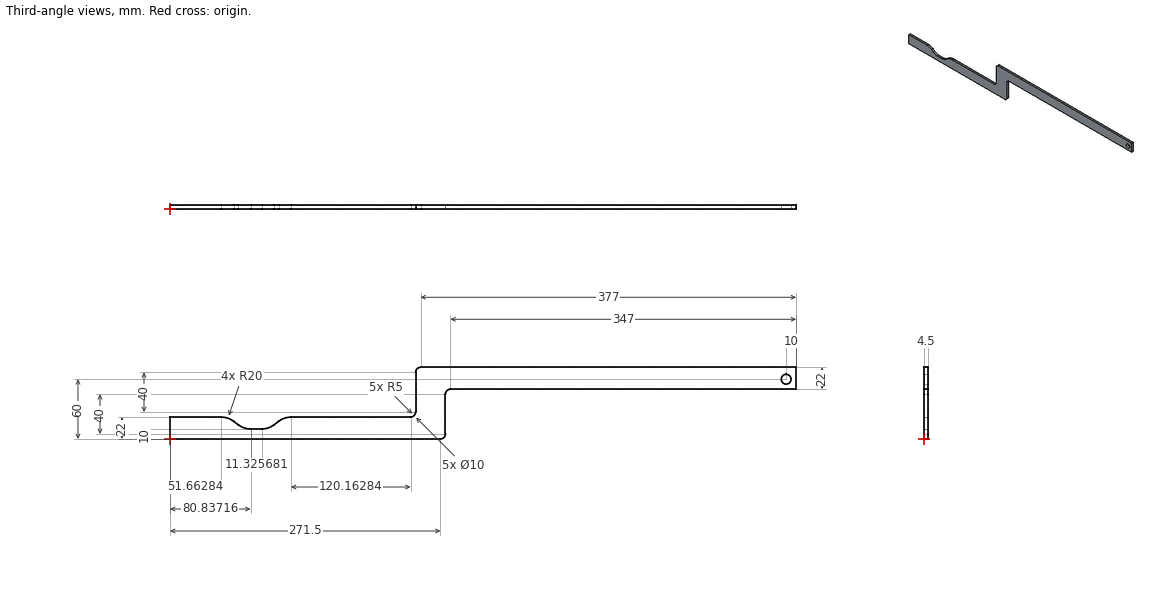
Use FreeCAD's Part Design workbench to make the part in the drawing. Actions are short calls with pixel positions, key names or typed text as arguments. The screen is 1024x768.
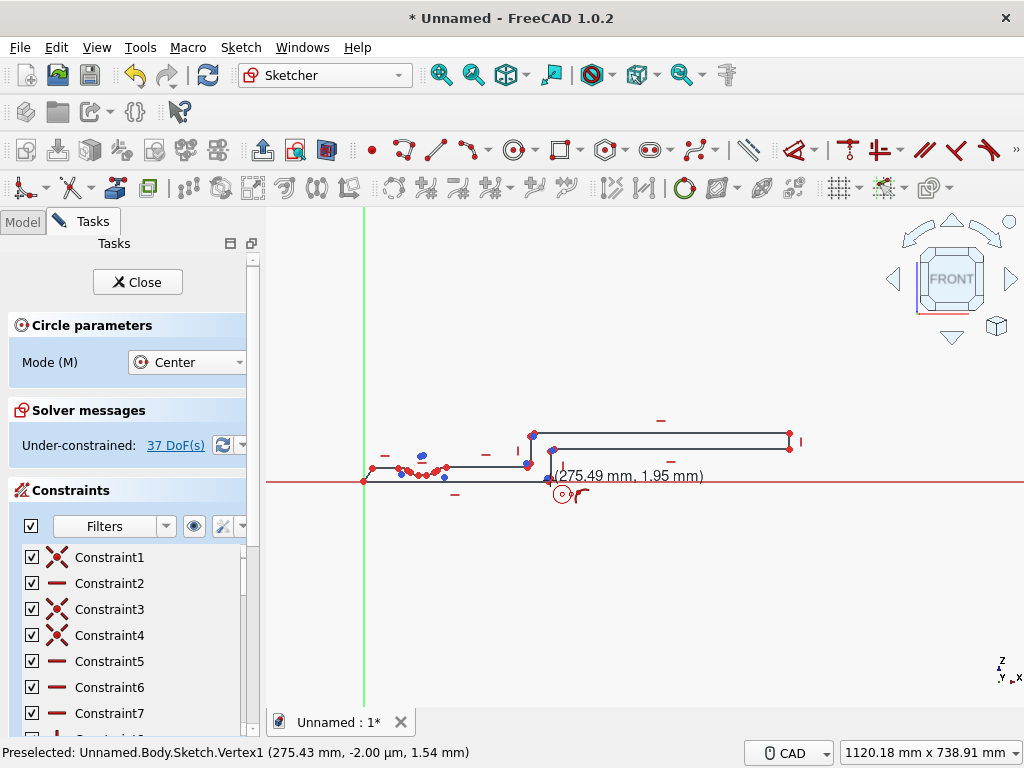
scroll(782, 441, up, 10)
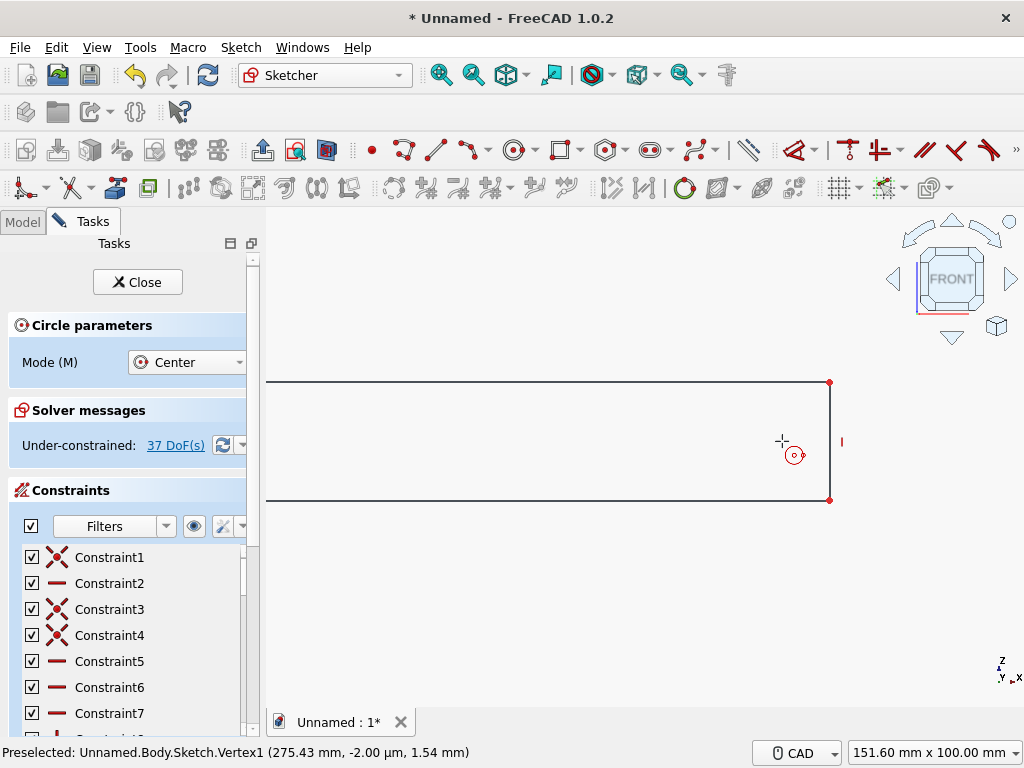
scroll(783, 441, down, 10)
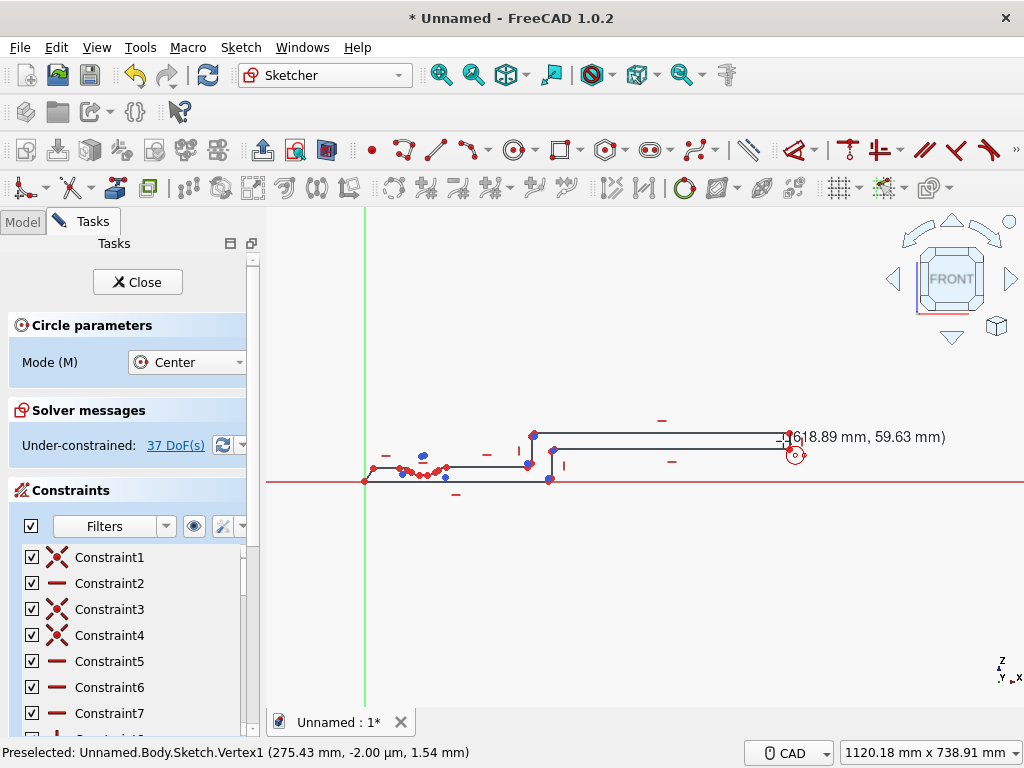
scroll(783, 441, up, 5)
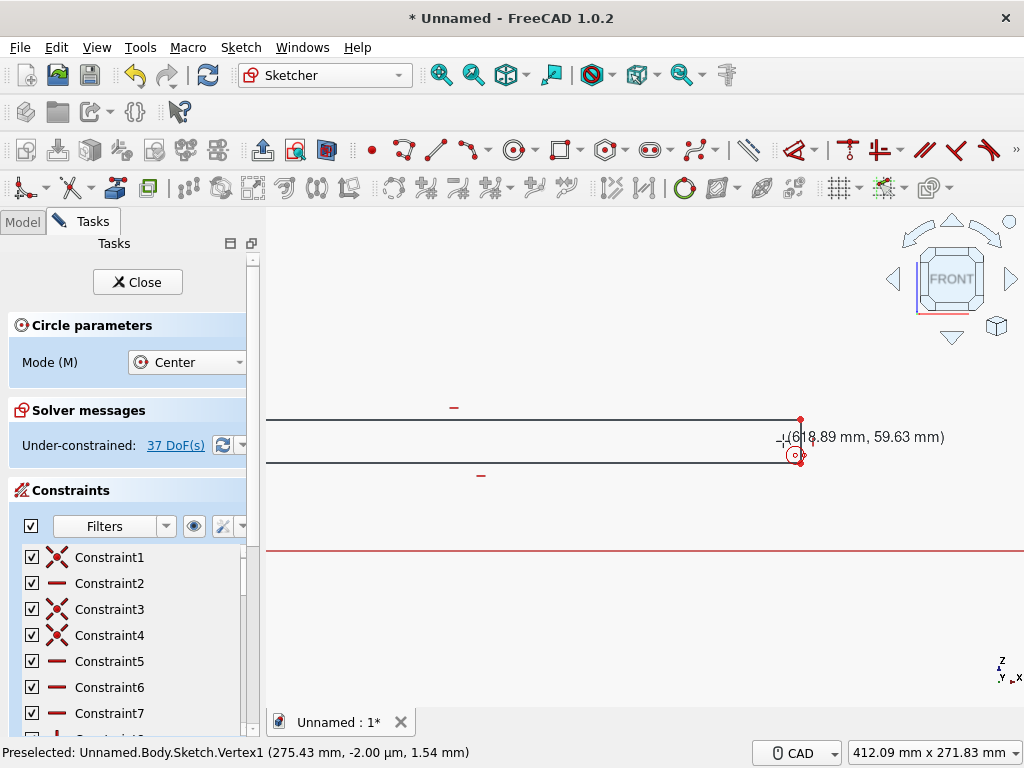
click(783, 441)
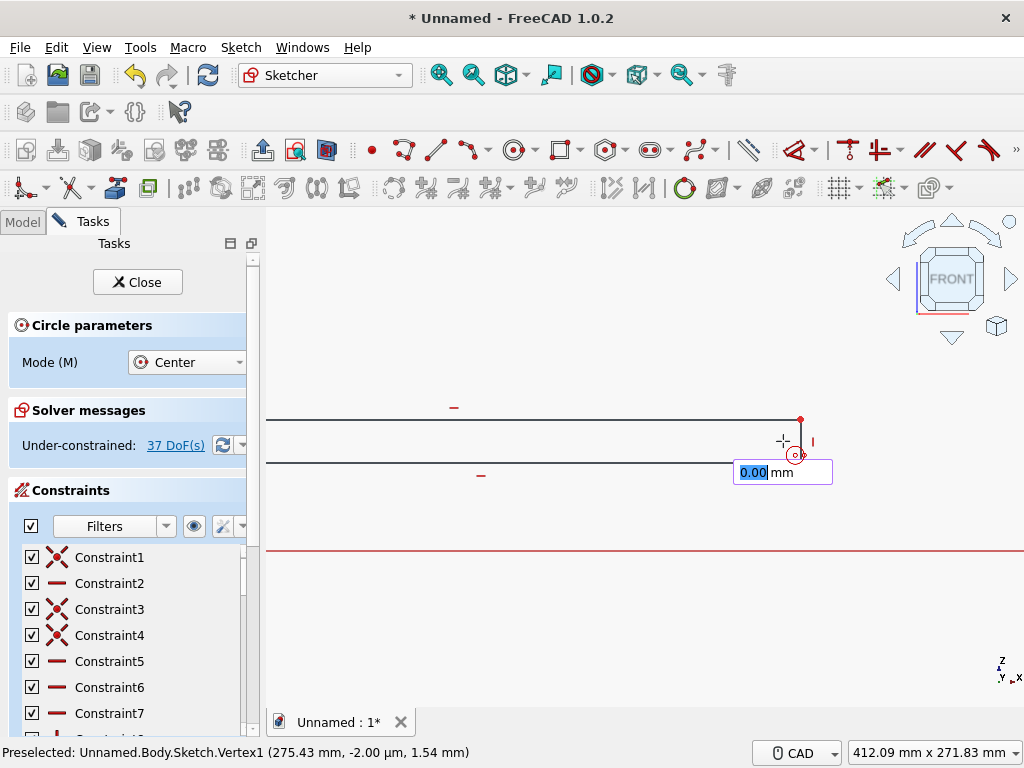
scroll(776, 434, up, 3)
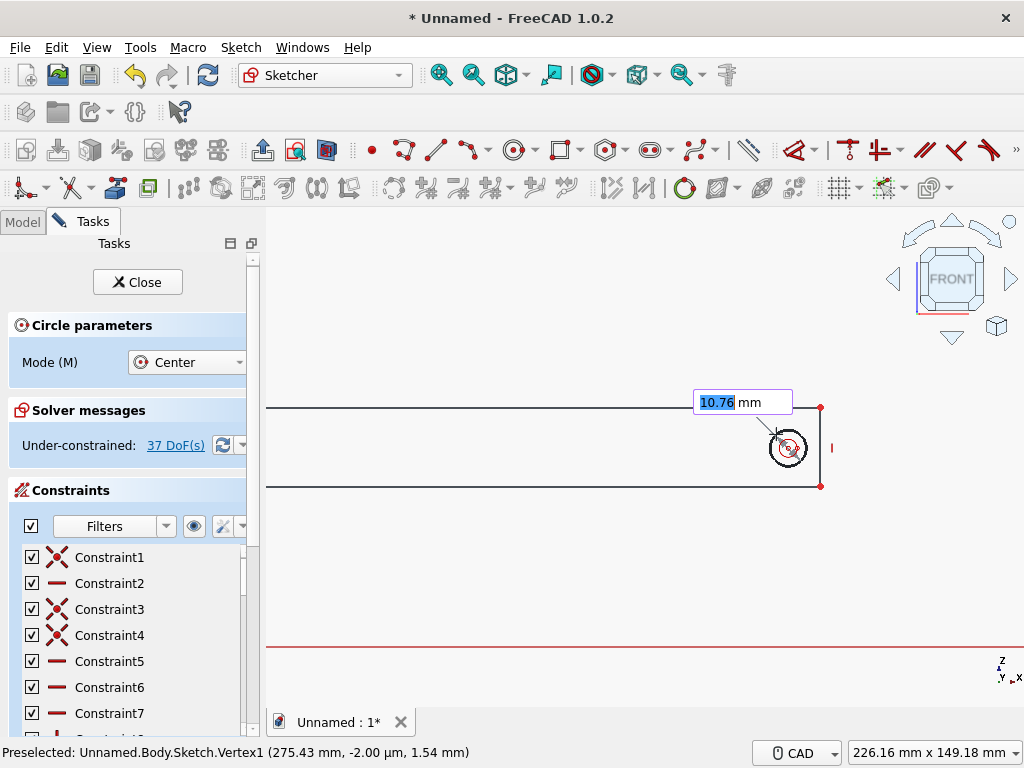
click(776, 435)
key(Escape)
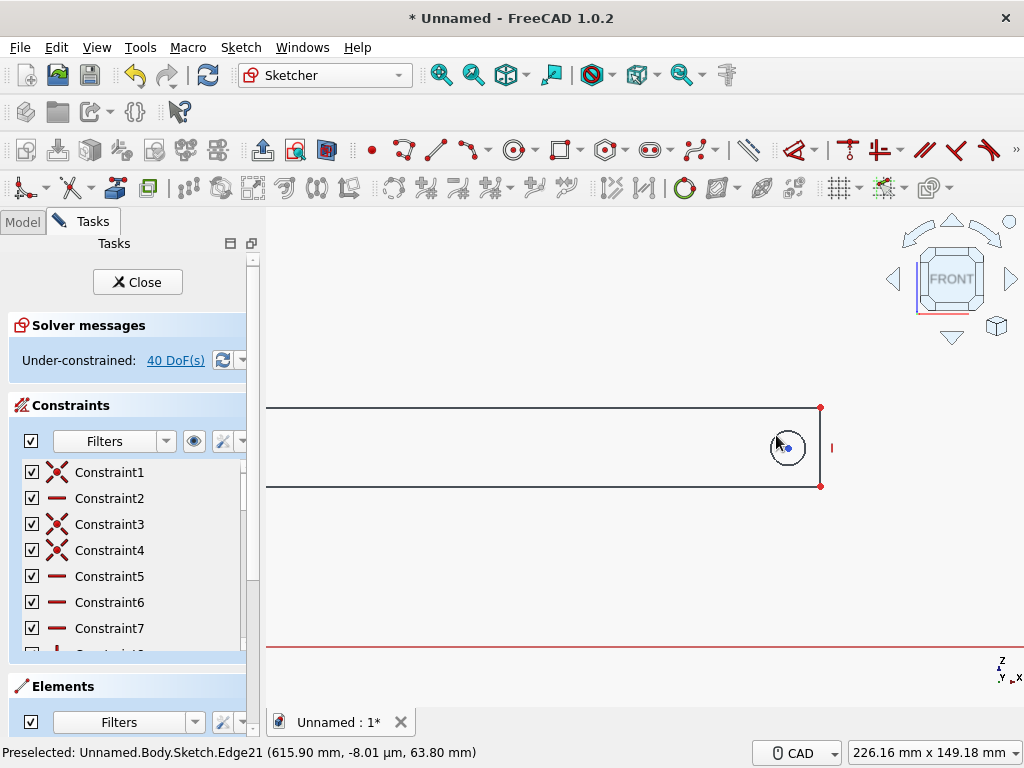
scroll(781, 439, down, 8)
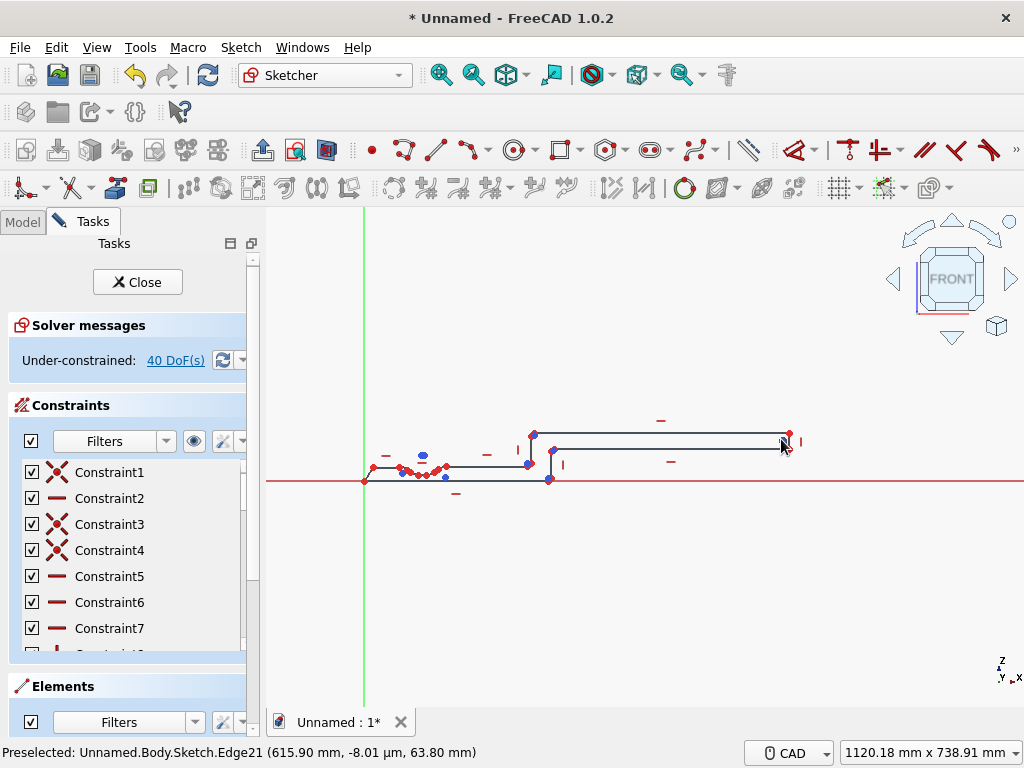
click(493, 481)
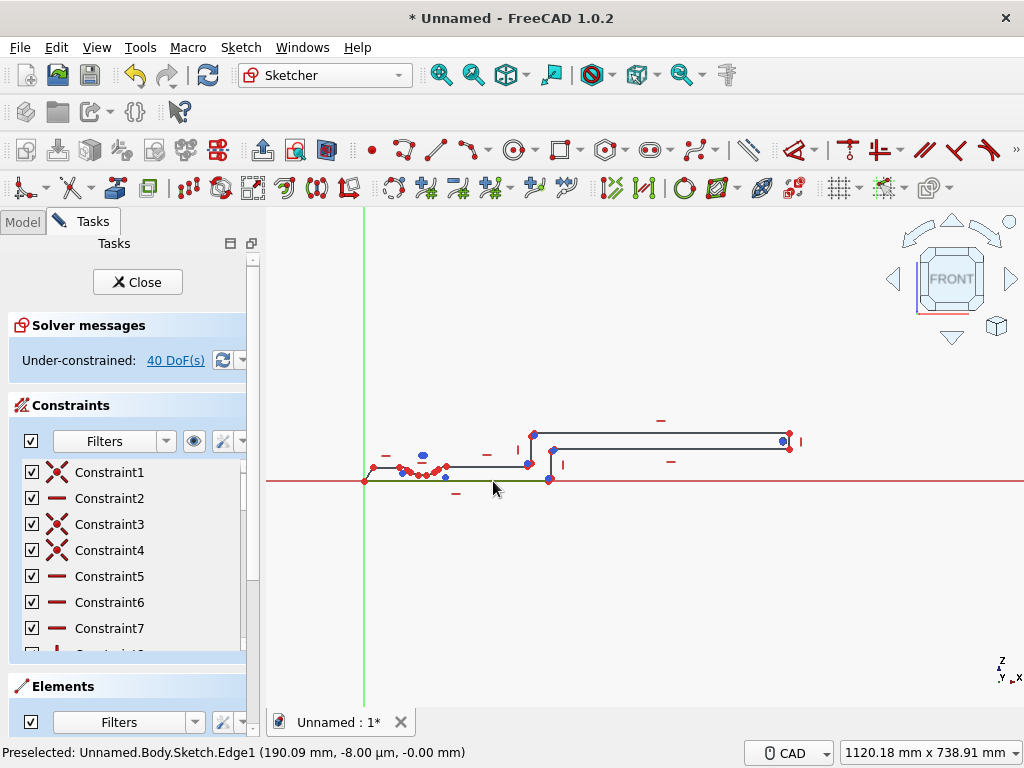
scroll(551, 481, up, 9)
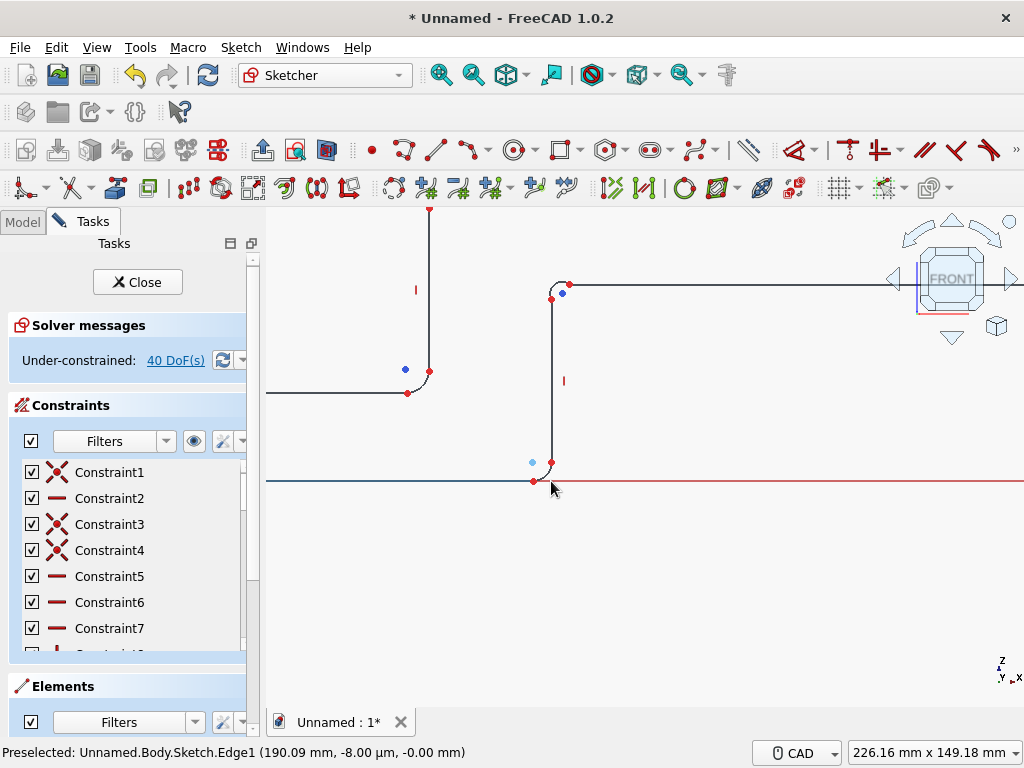
click(546, 475)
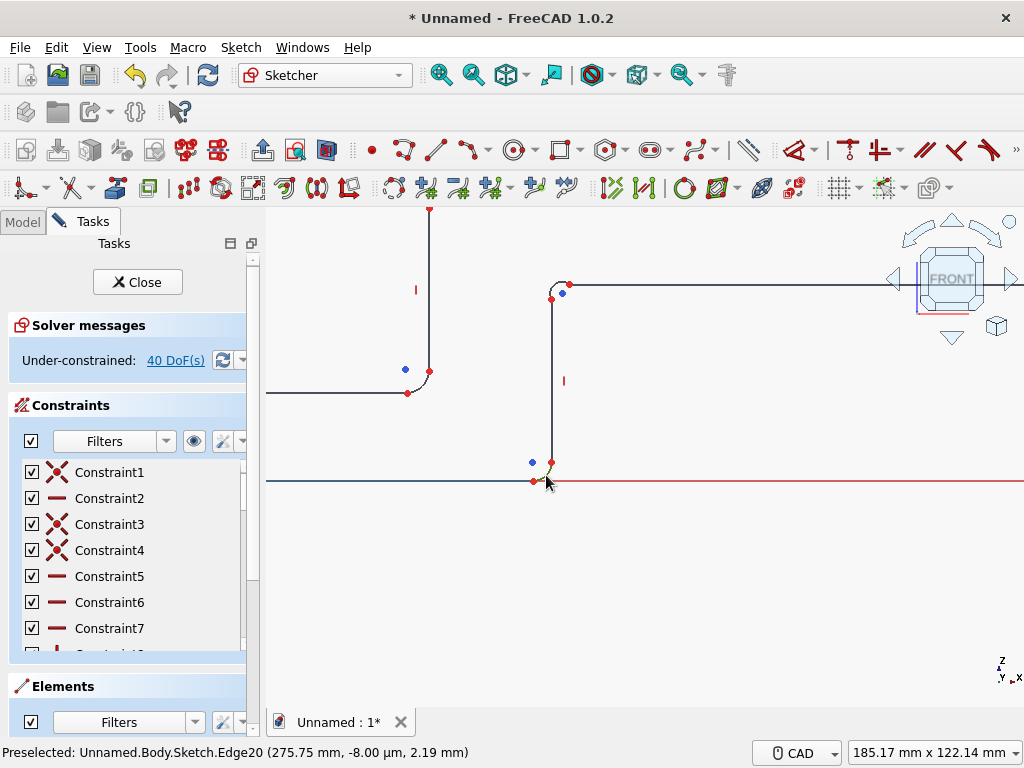
key(t)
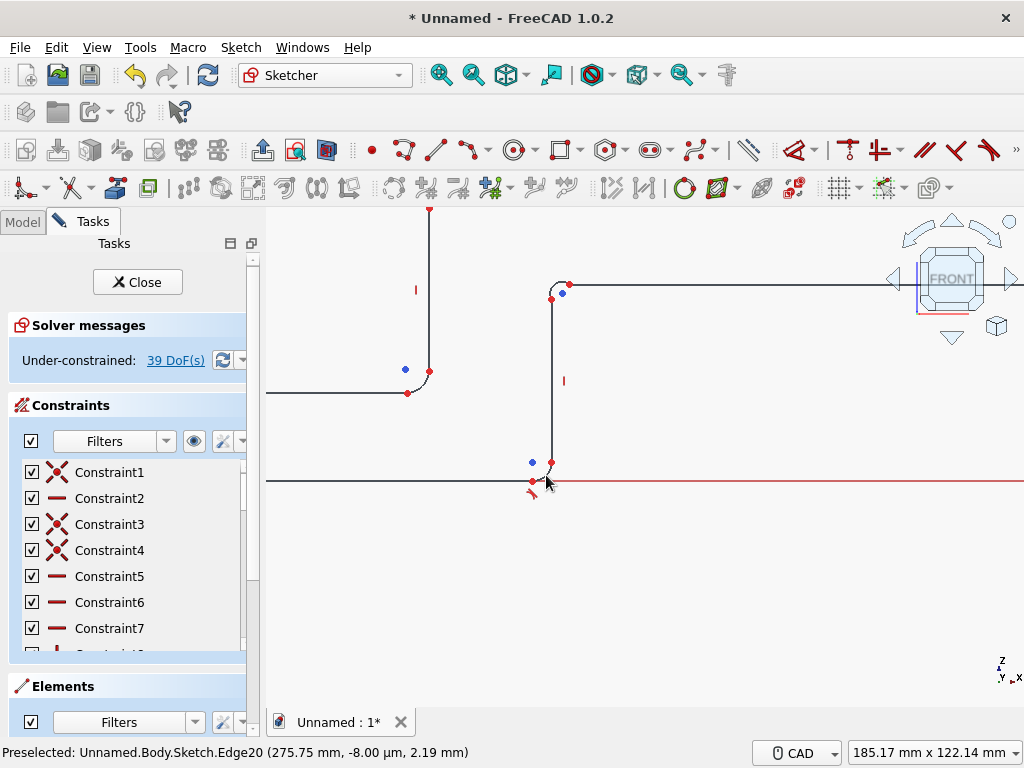
scroll(551, 481, down, 9)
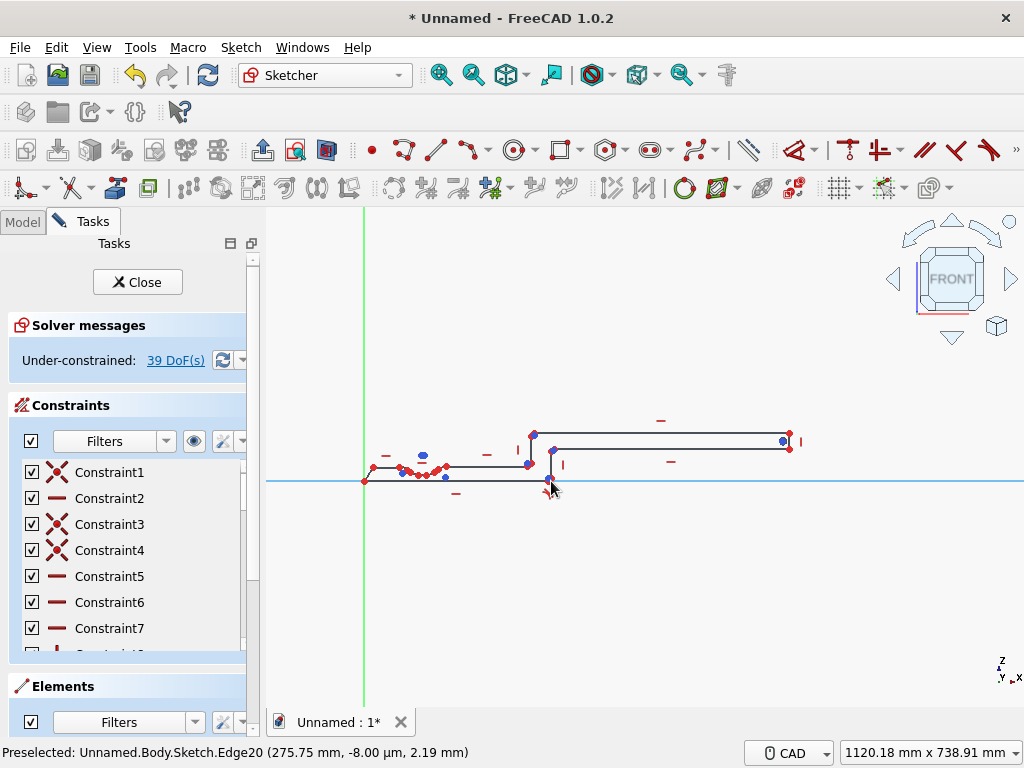
scroll(381, 468, up, 3)